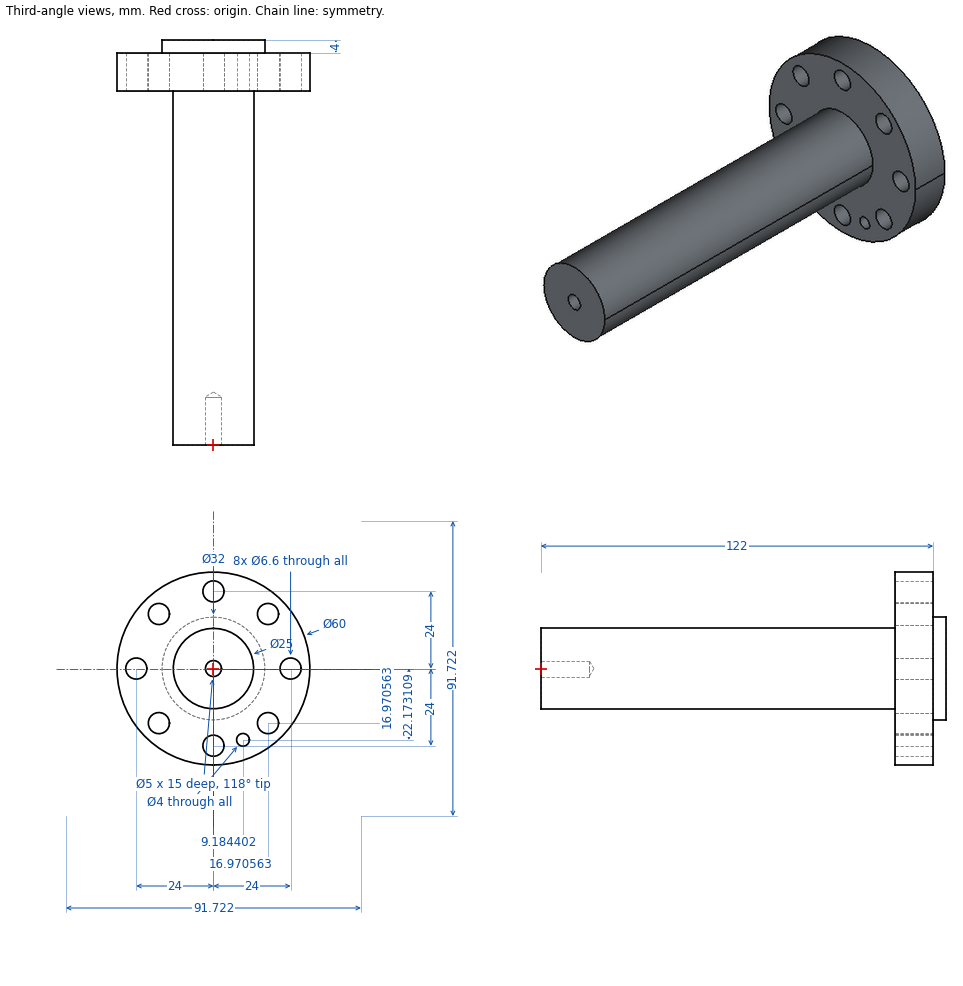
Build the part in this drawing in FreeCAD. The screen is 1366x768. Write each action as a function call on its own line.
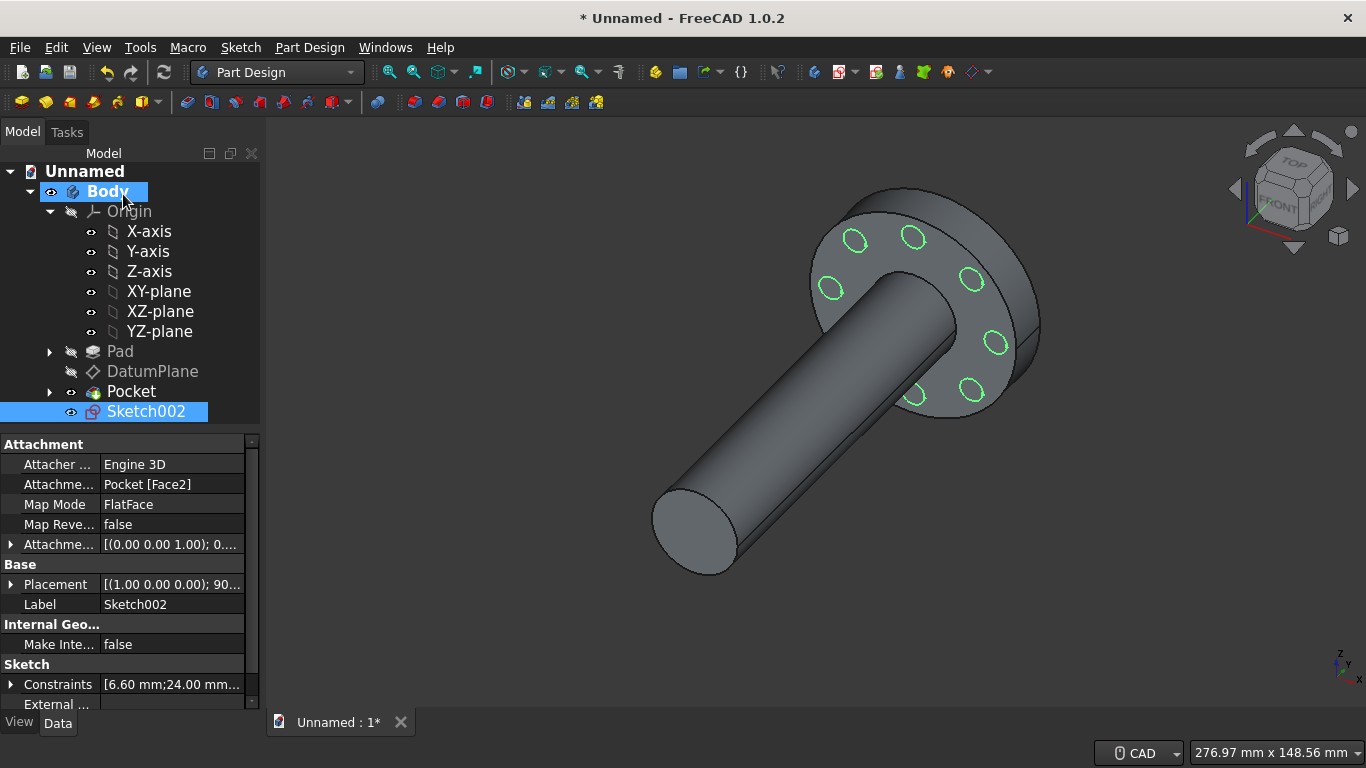
click(212, 102)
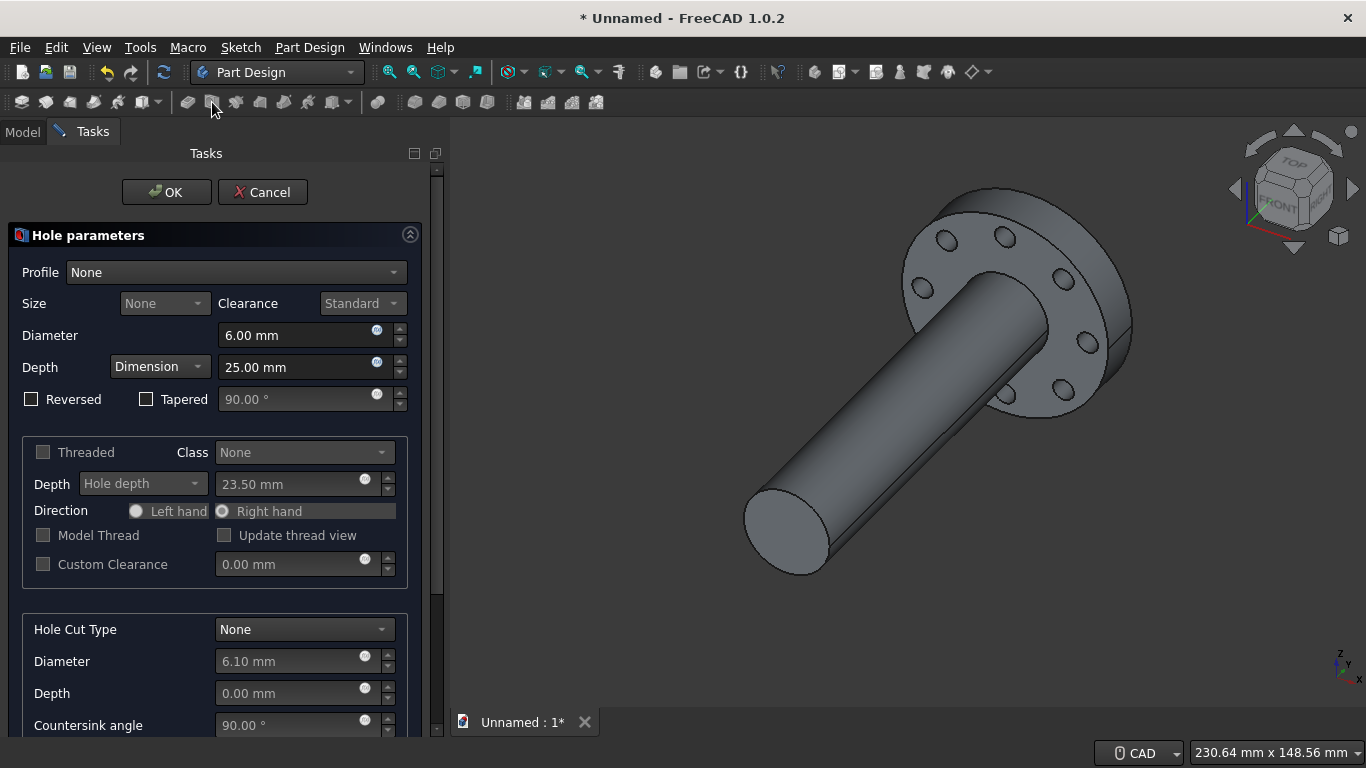
triple_click(305, 335)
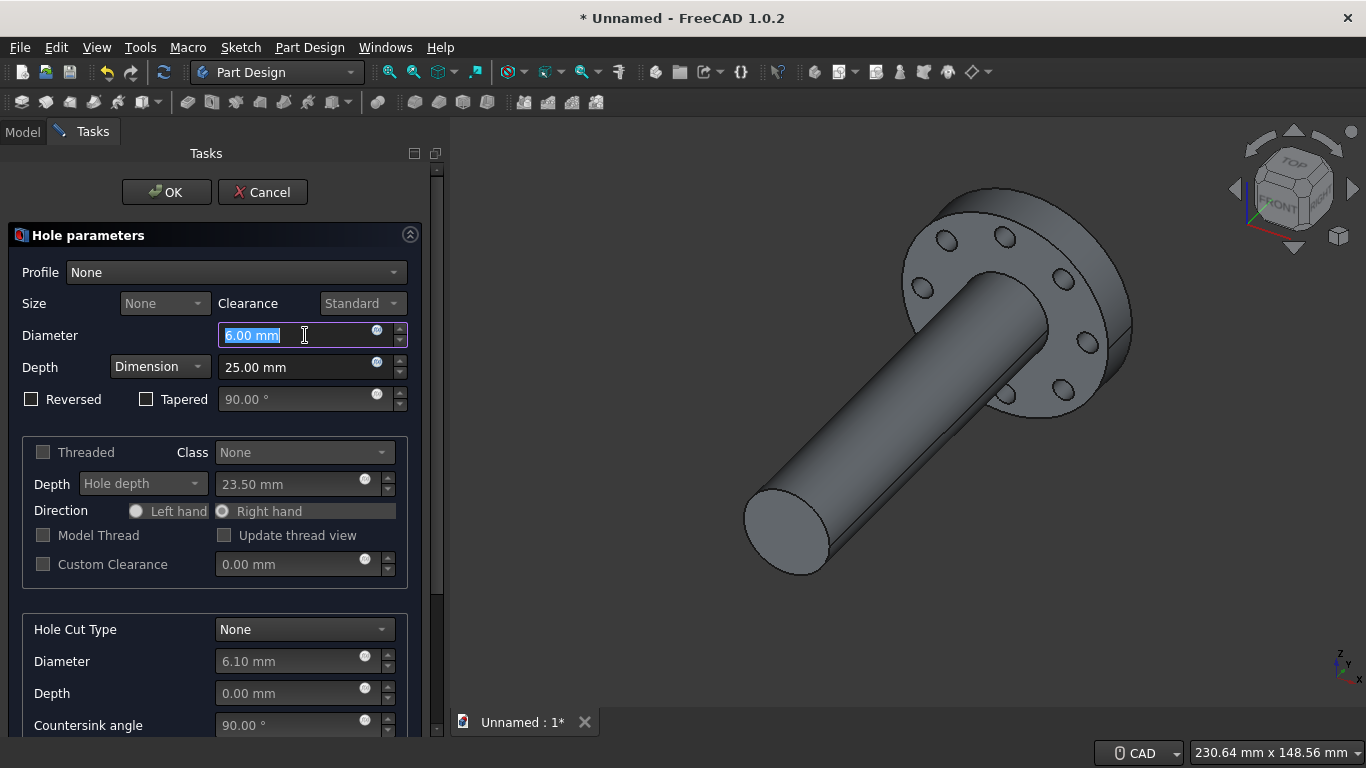
text(6.6)
key(Tab)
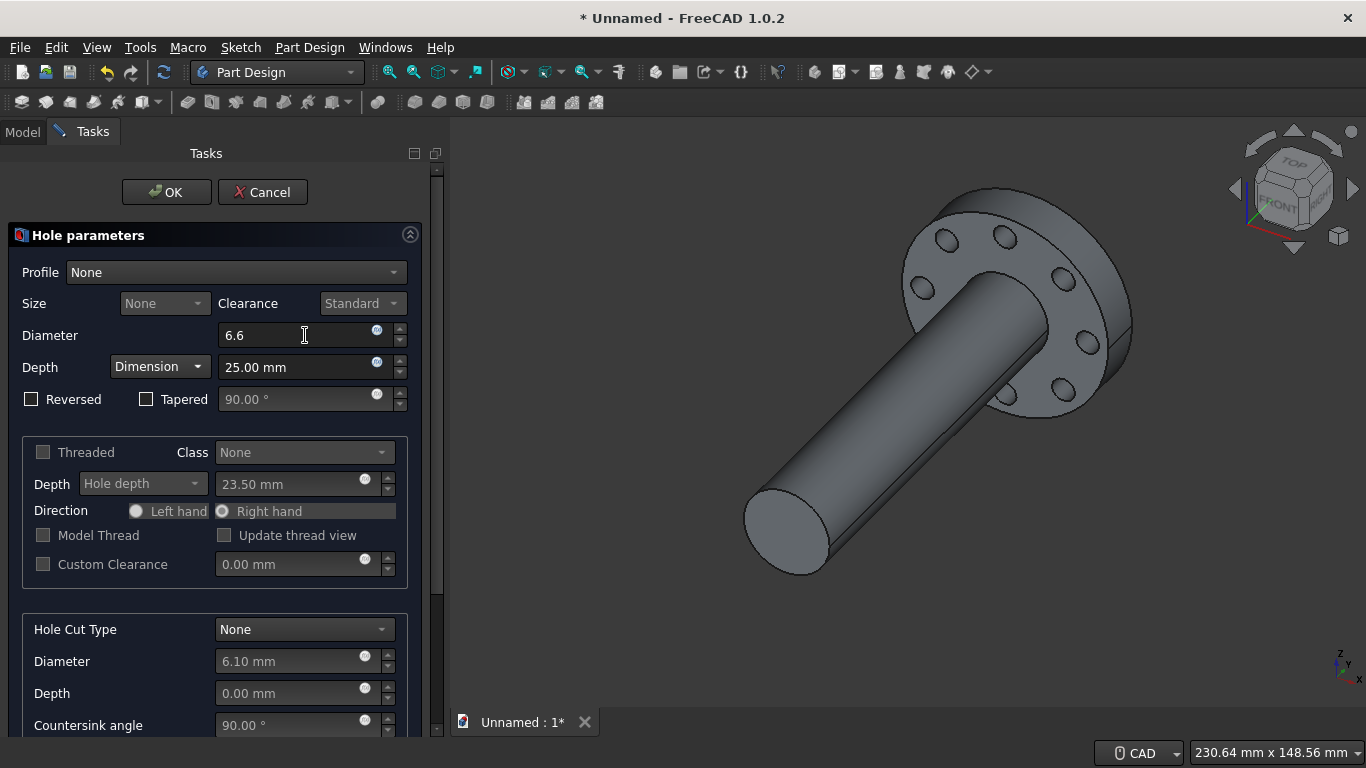
click(161, 366)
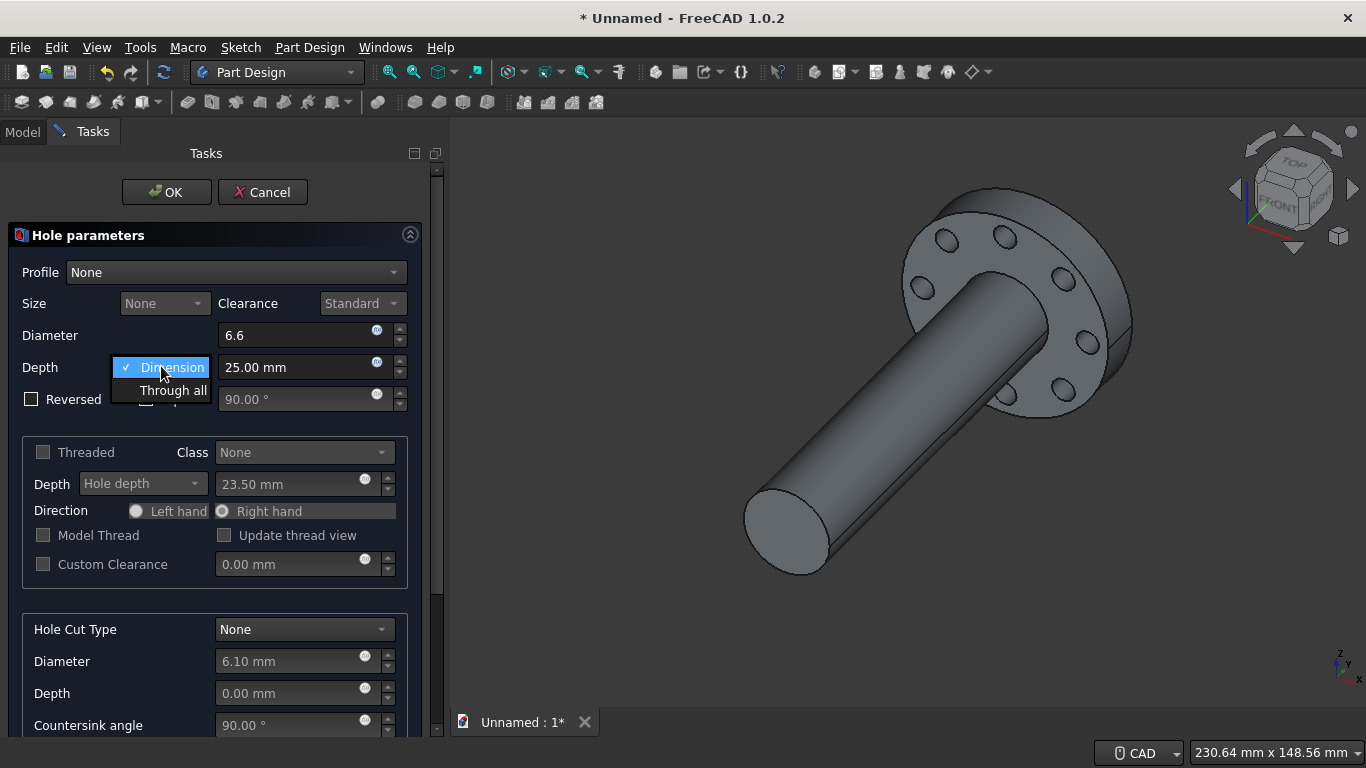
click(160, 390)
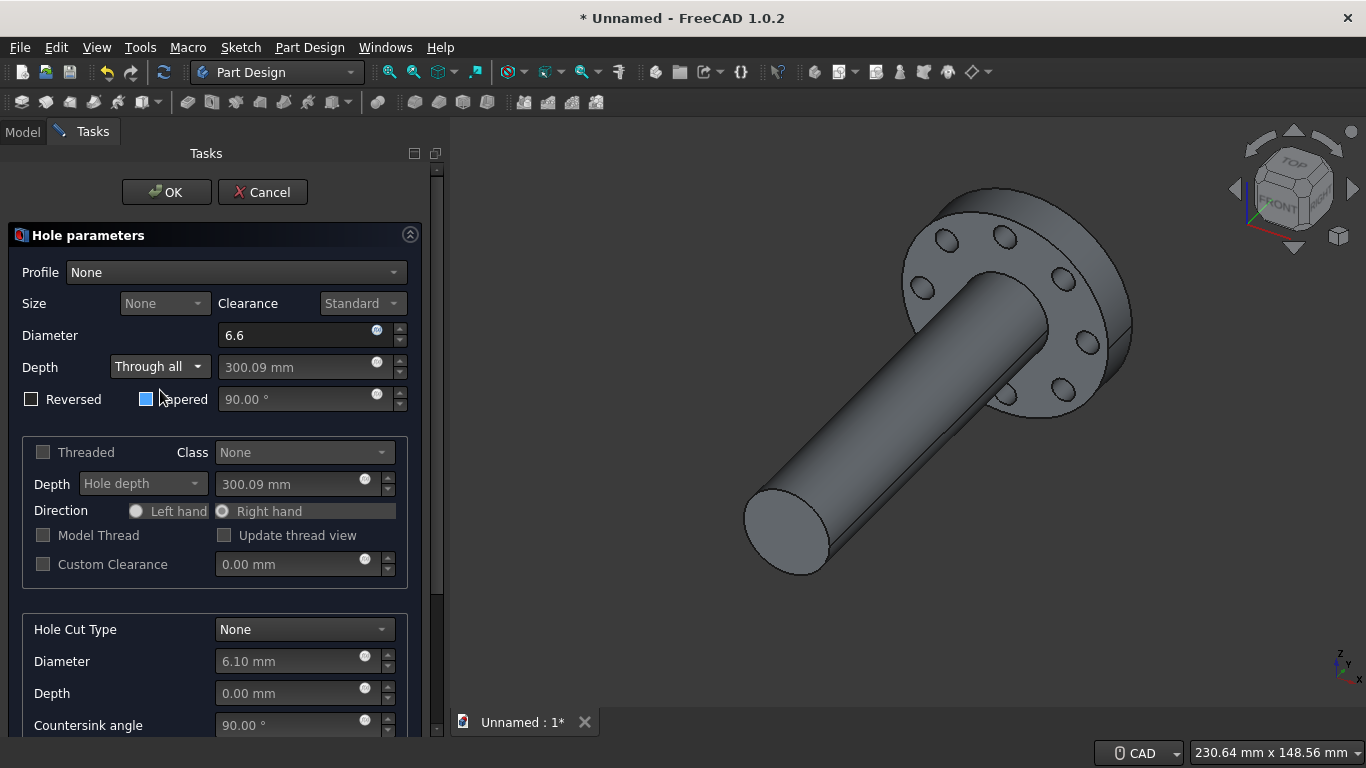
click(167, 192)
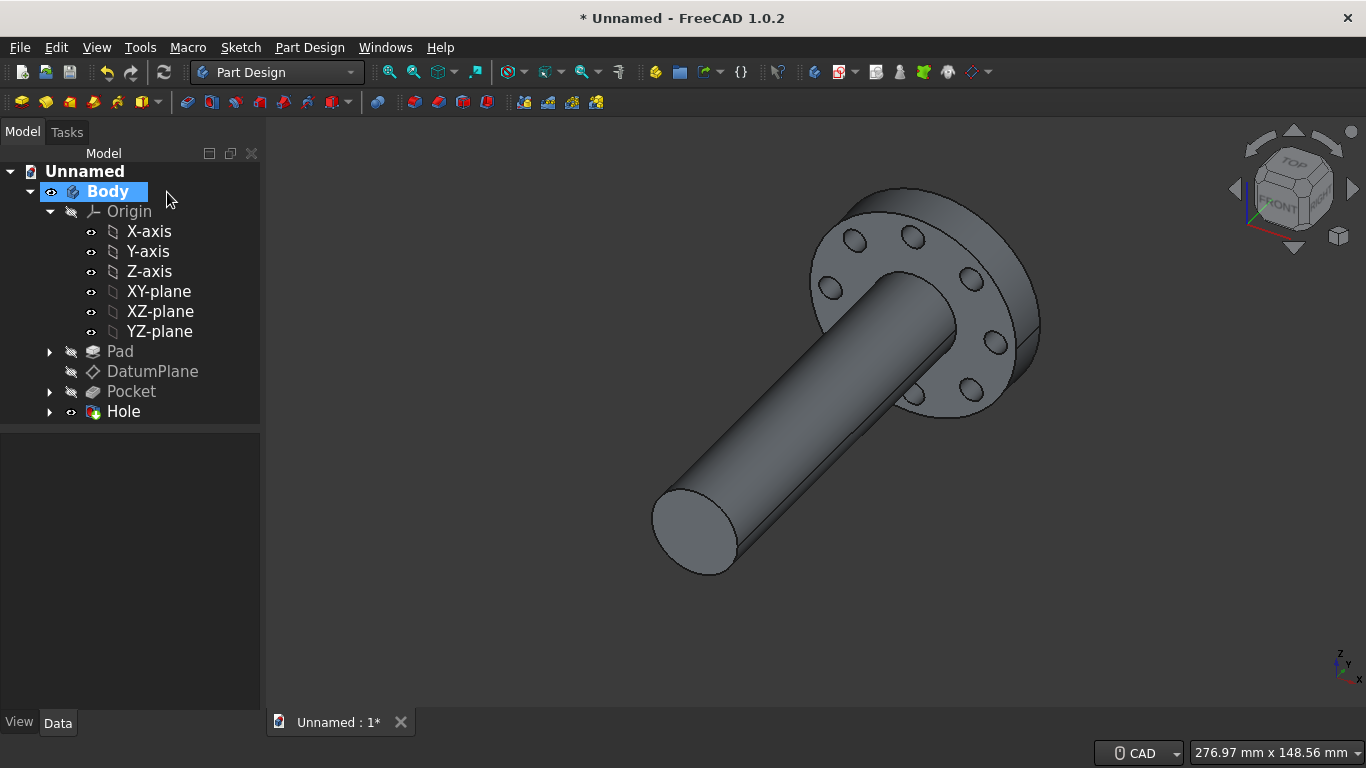
key(4)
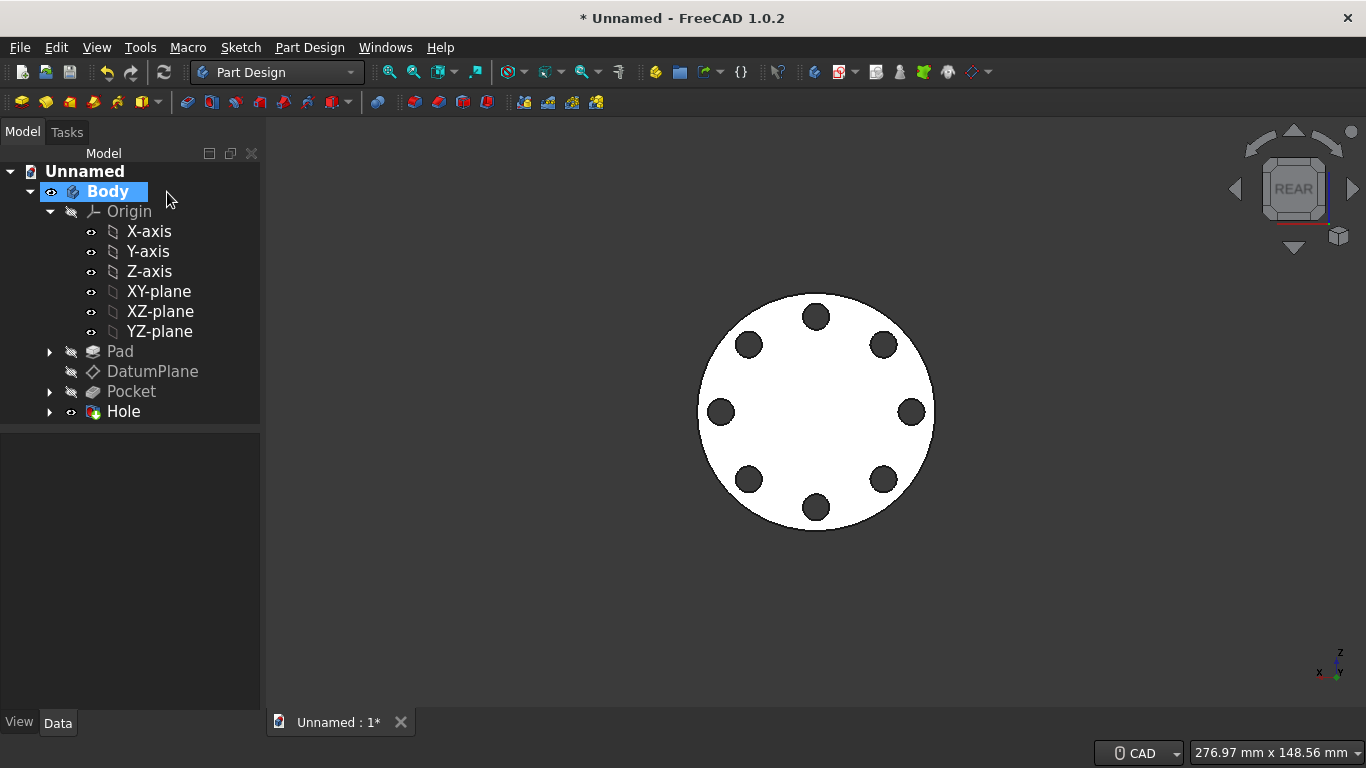
key(v)
key(f)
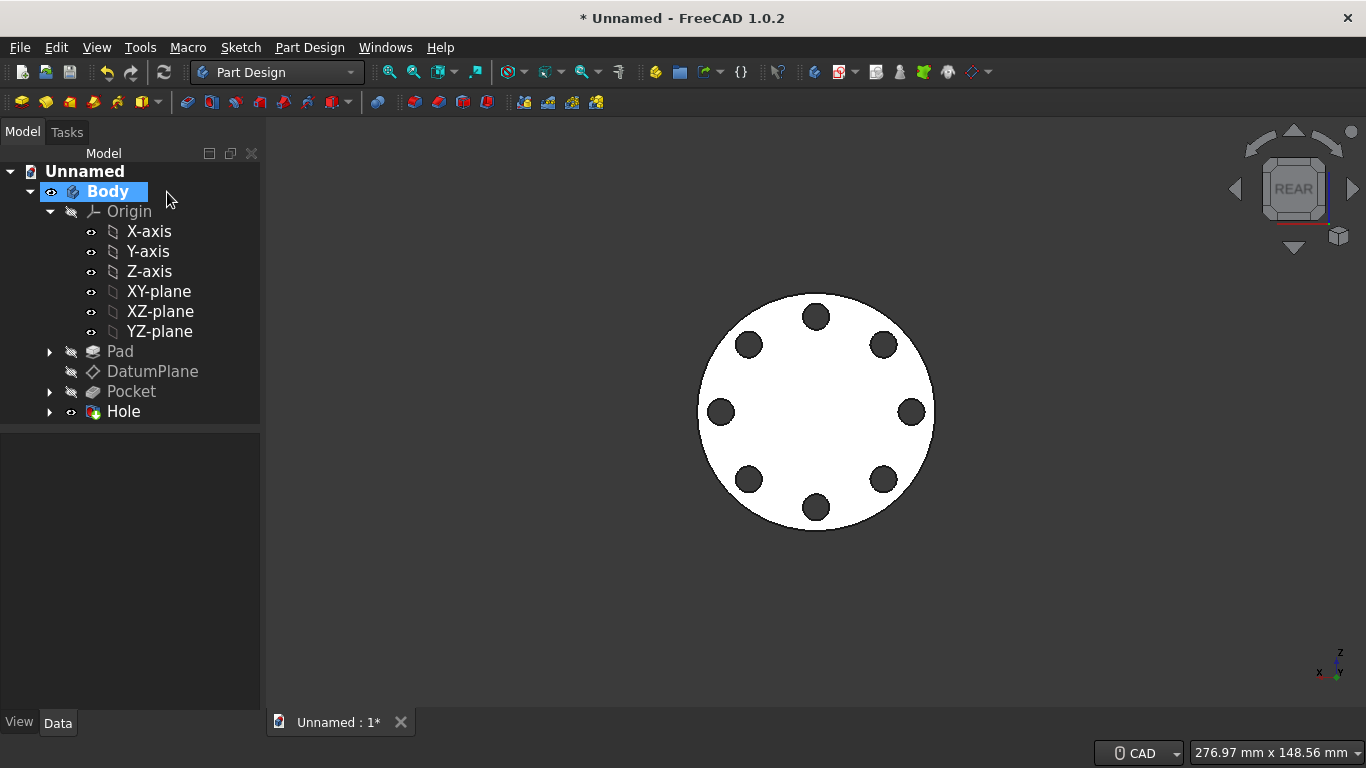
click(816, 411)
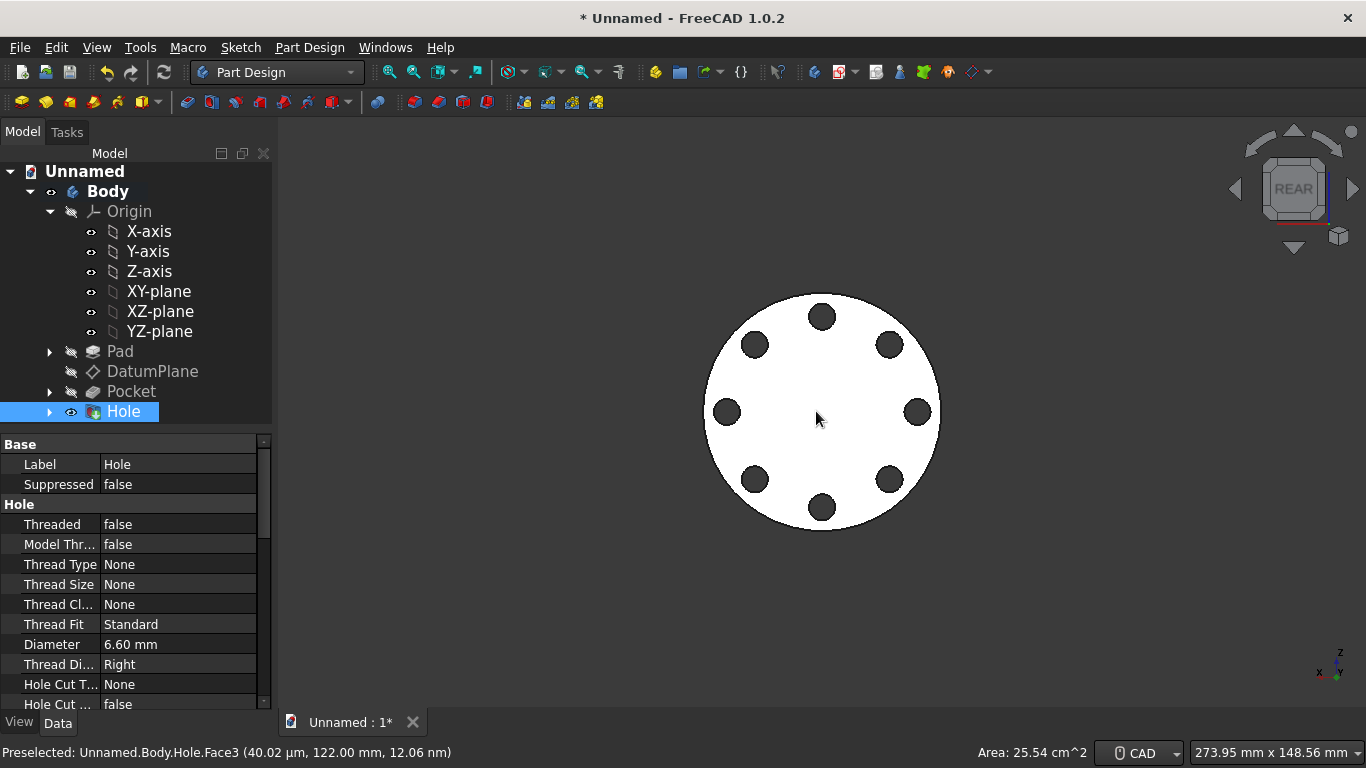
click(840, 72)